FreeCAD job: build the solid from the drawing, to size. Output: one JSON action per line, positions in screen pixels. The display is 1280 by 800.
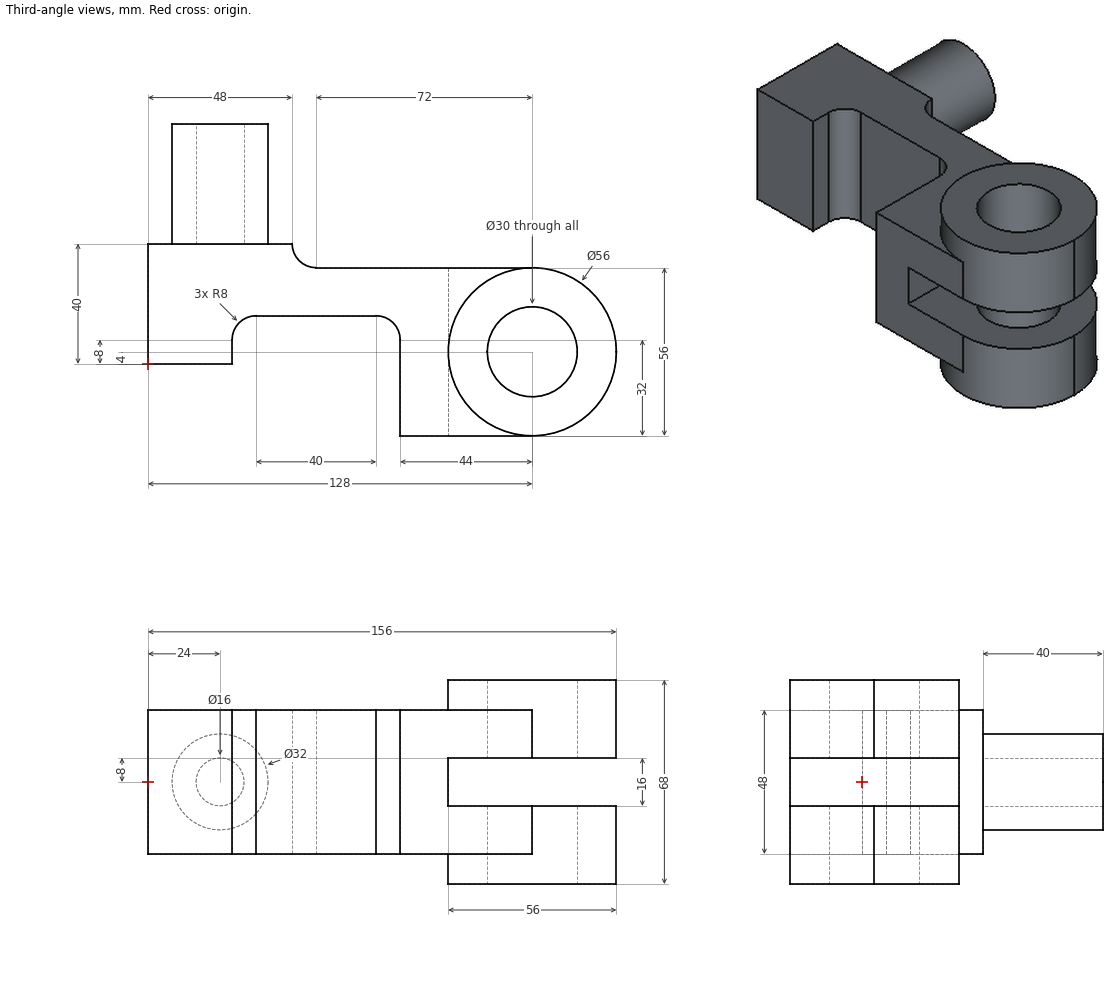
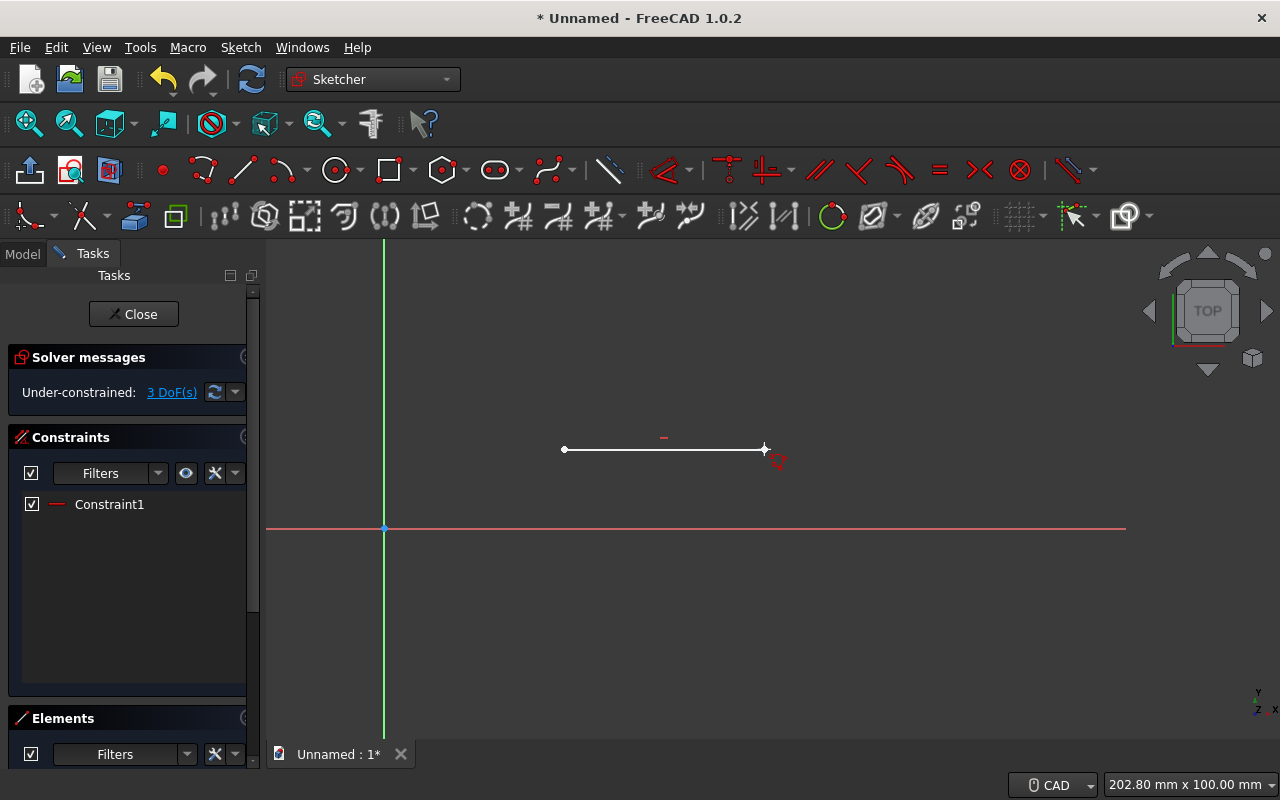
{"action": "left_click", "coordinate": [804, 489]}
{"action": "left_click", "coordinate": [804, 649]}
{"action": "left_click", "coordinate": [1024, 649]}
{"action": "left_click", "coordinate": [1024, 369]}
{"action": "left_click", "coordinate": [664, 369]}
{"action": "right_click", "coordinate": [664, 369]}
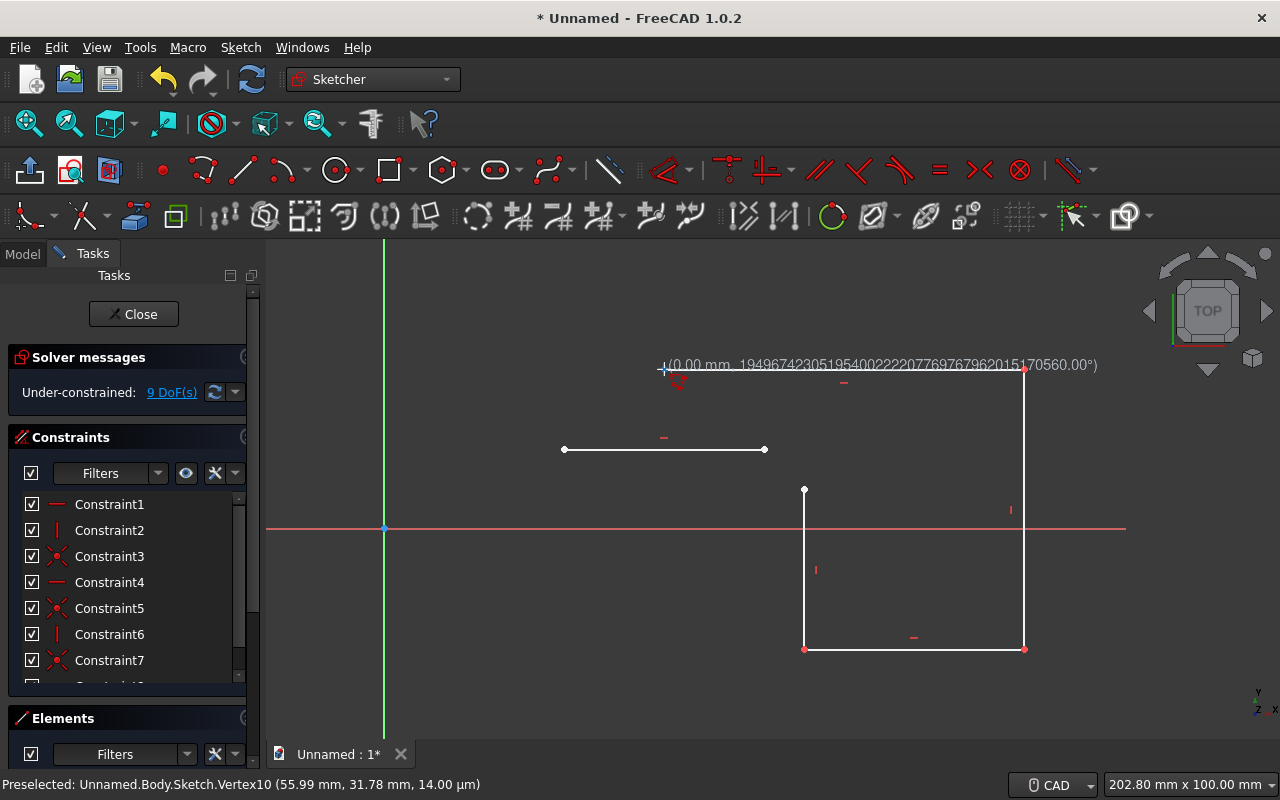
{"action": "left_click", "coordinate": [624, 329]}
{"action": "left_click", "coordinate": [384, 329]}
{"action": "left_click", "coordinate": [384, 529]}
{"action": "left_click", "coordinate": [524, 520]}
{"action": "left_click", "coordinate": [524, 489]}
{"action": "right_click", "coordinate": [524, 489]}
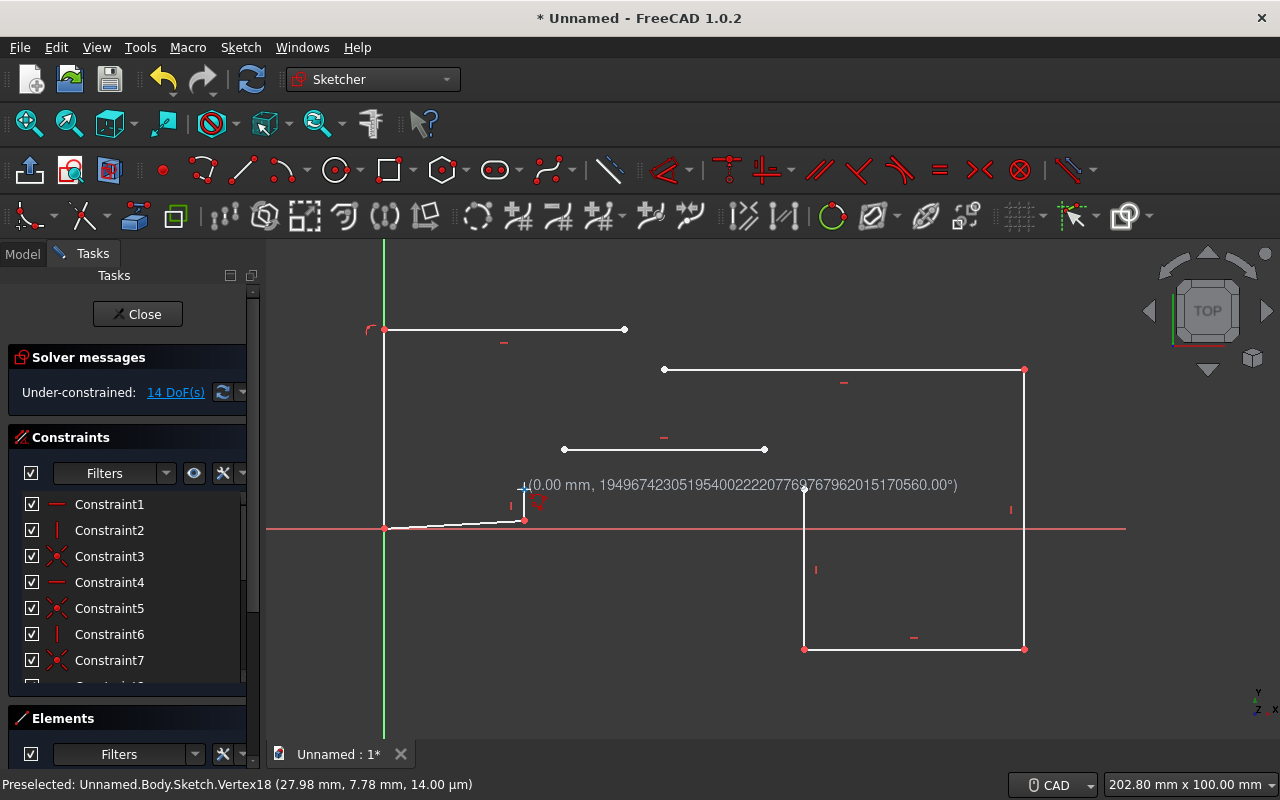
{"action": "key", "text": "g 3 a"}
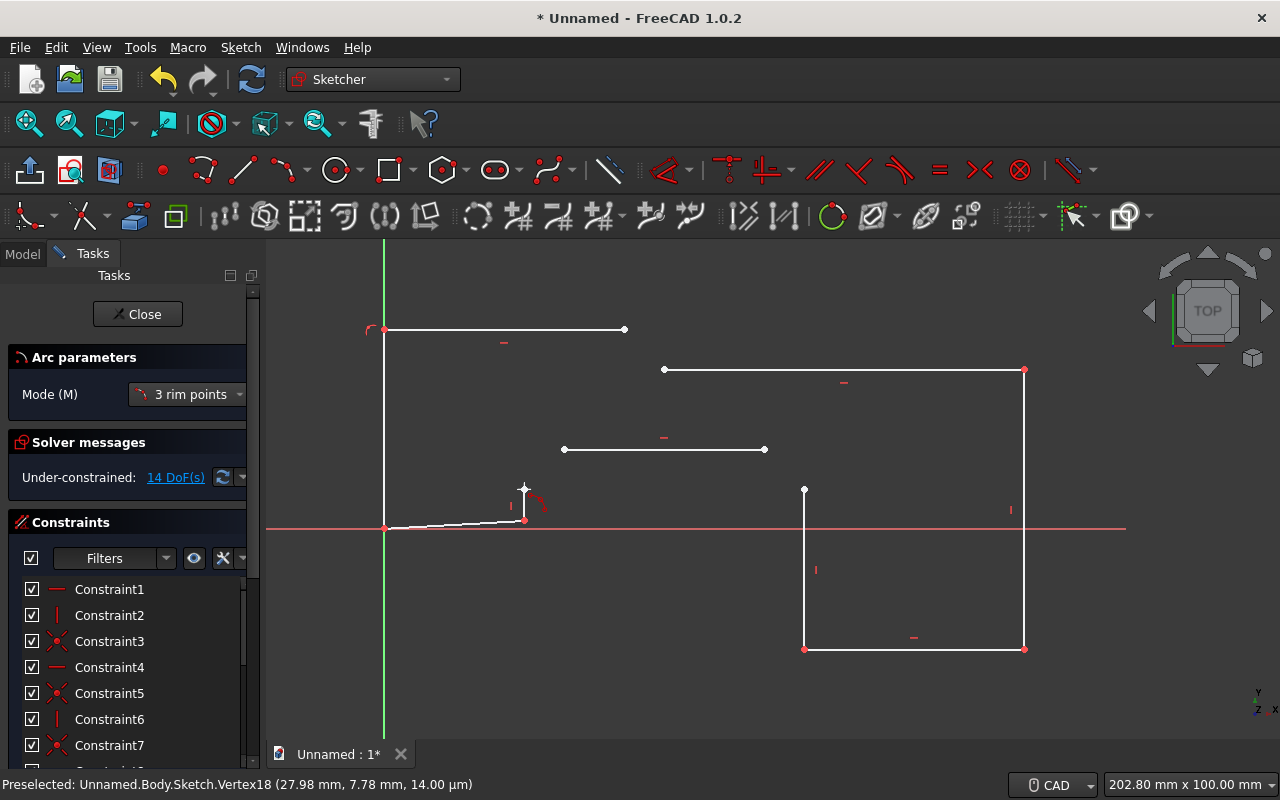
{"action": "left_click", "coordinate": [764, 450]}
{"action": "left_click", "coordinate": [804, 490]}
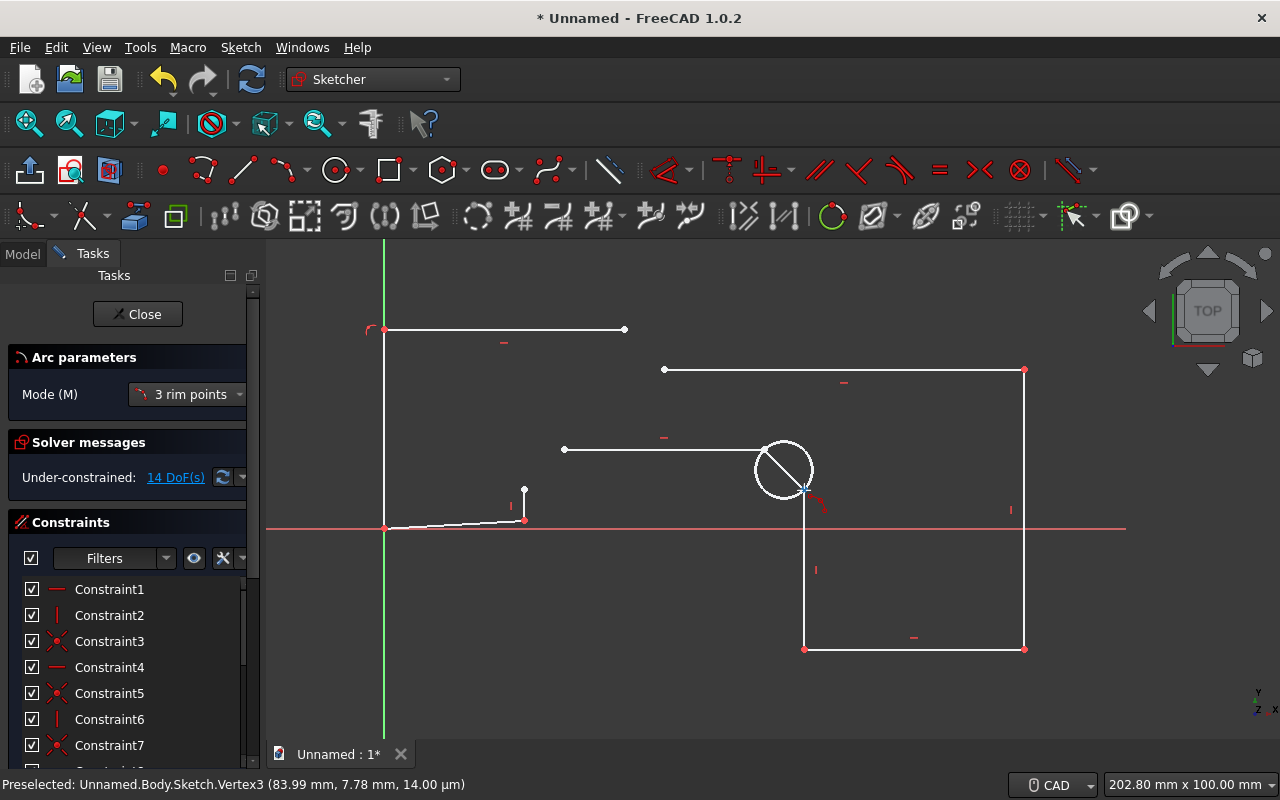
{"action": "scroll", "coordinate": [792, 461], "scroll_direction": "up", "scroll_amount": 2}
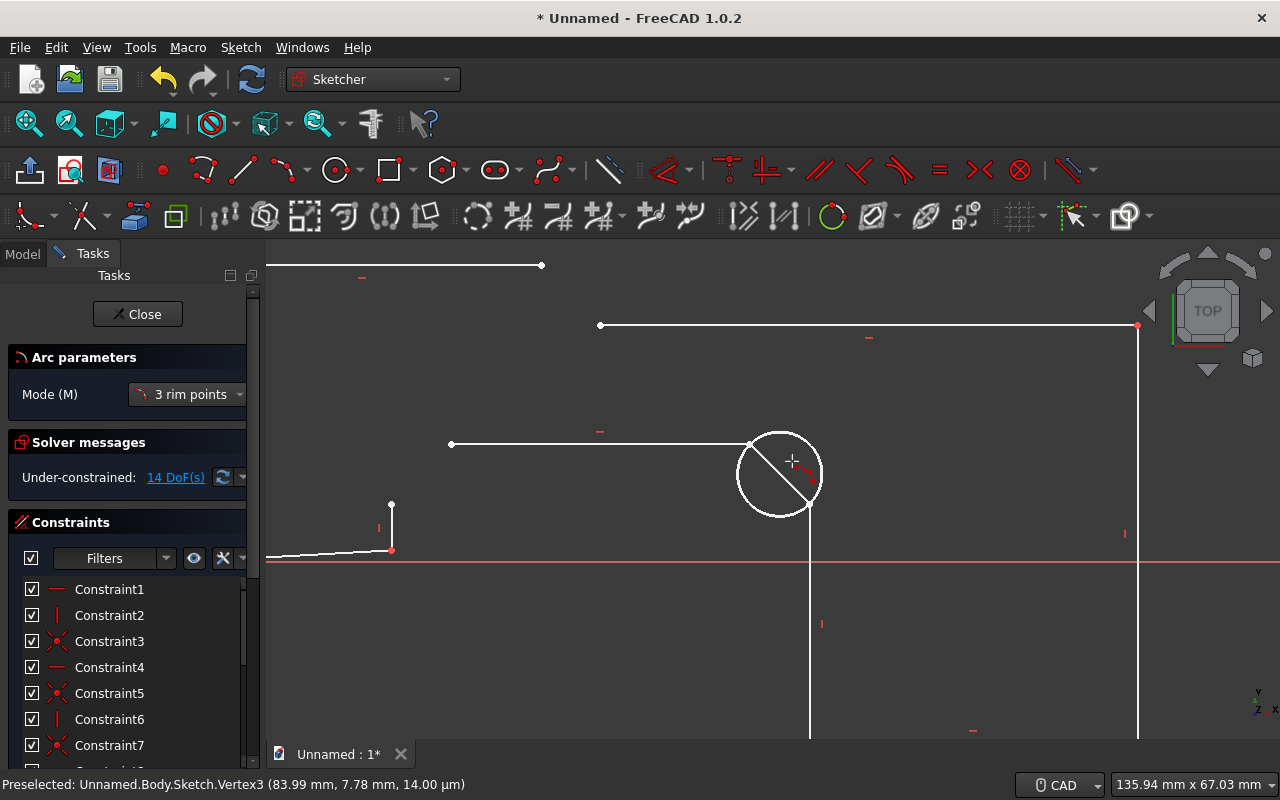
{"action": "left_click", "coordinate": [792, 460]}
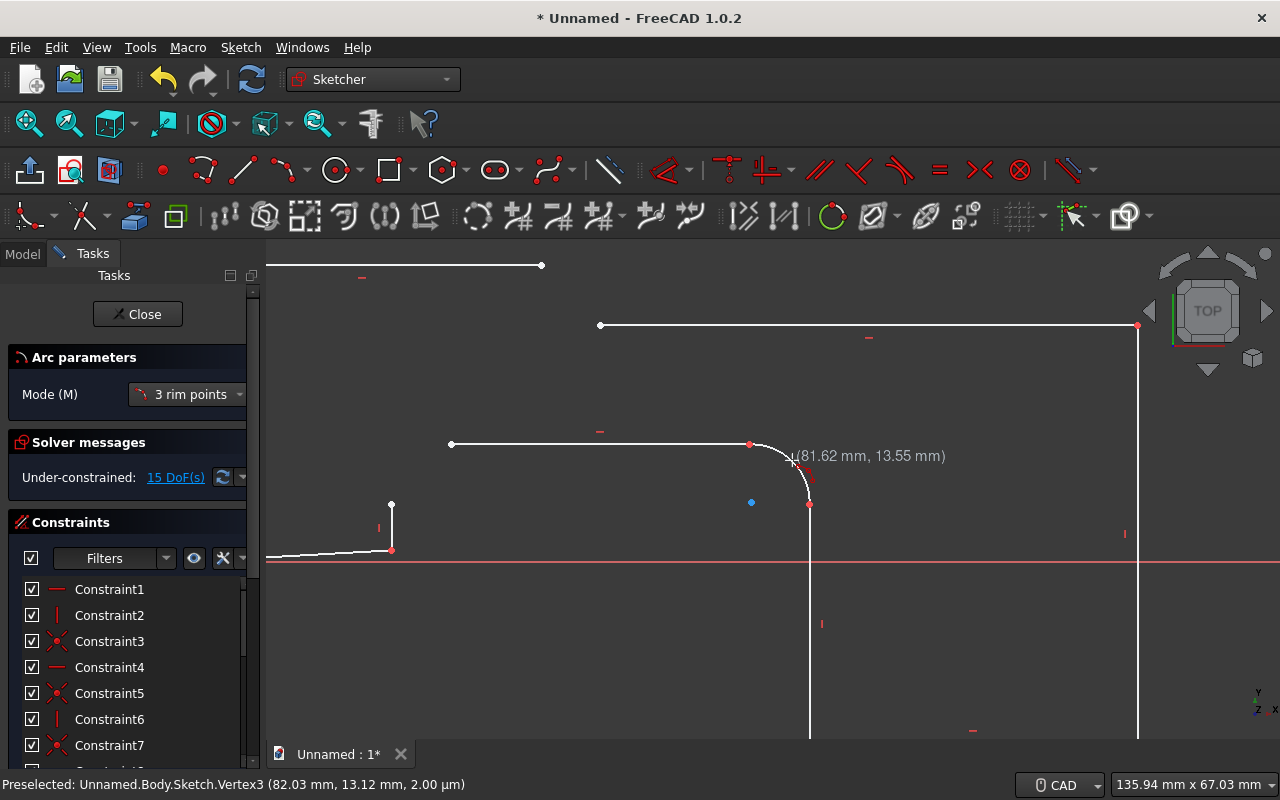
{"action": "left_click", "coordinate": [601, 325]}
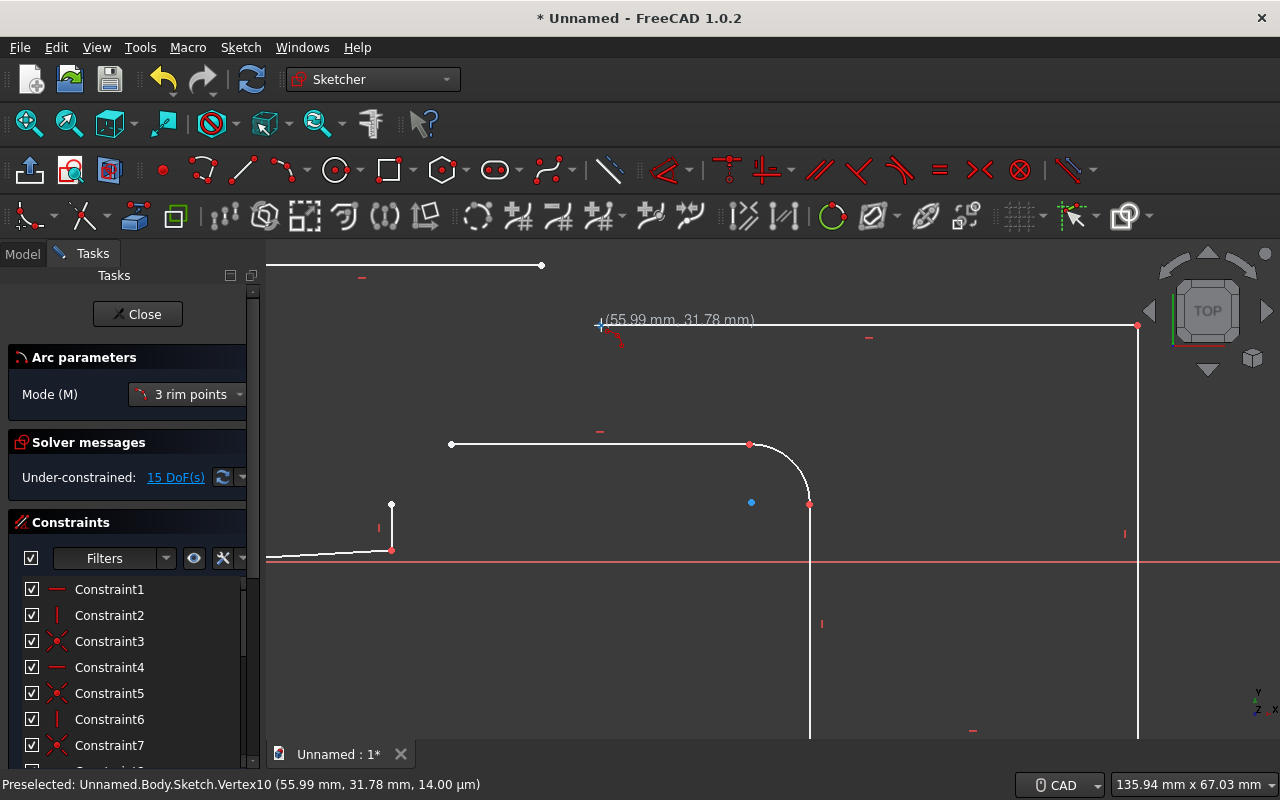
{"action": "scroll", "coordinate": [794, 462], "scroll_direction": "down", "scroll_amount": 2}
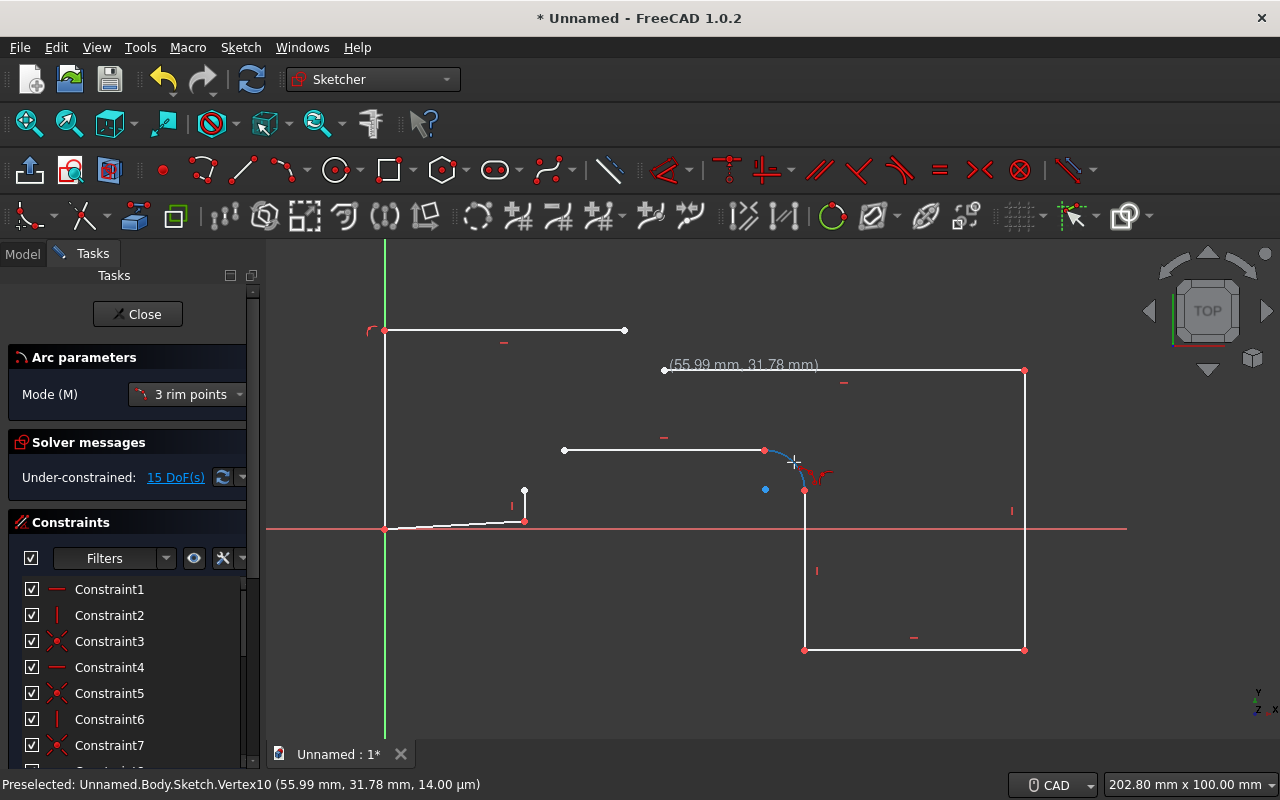
{"action": "left_click", "coordinate": [625, 330]}